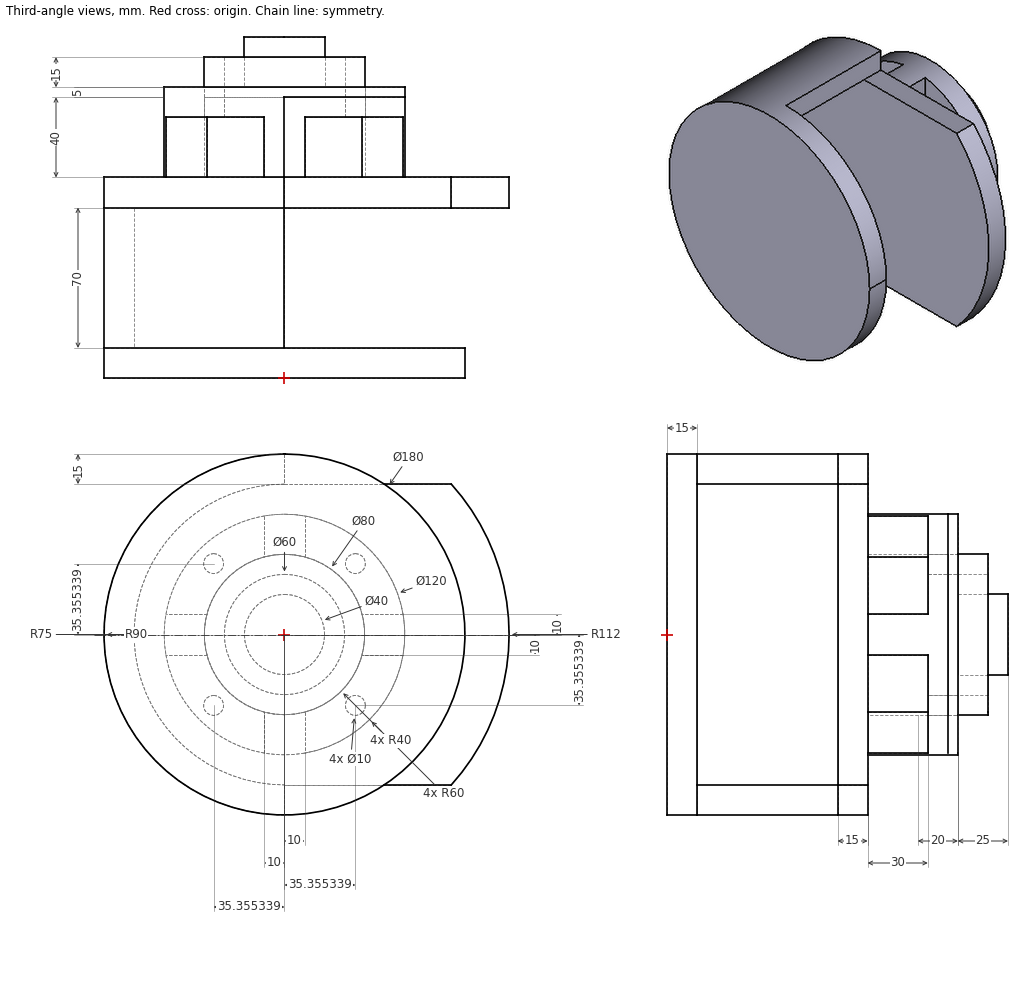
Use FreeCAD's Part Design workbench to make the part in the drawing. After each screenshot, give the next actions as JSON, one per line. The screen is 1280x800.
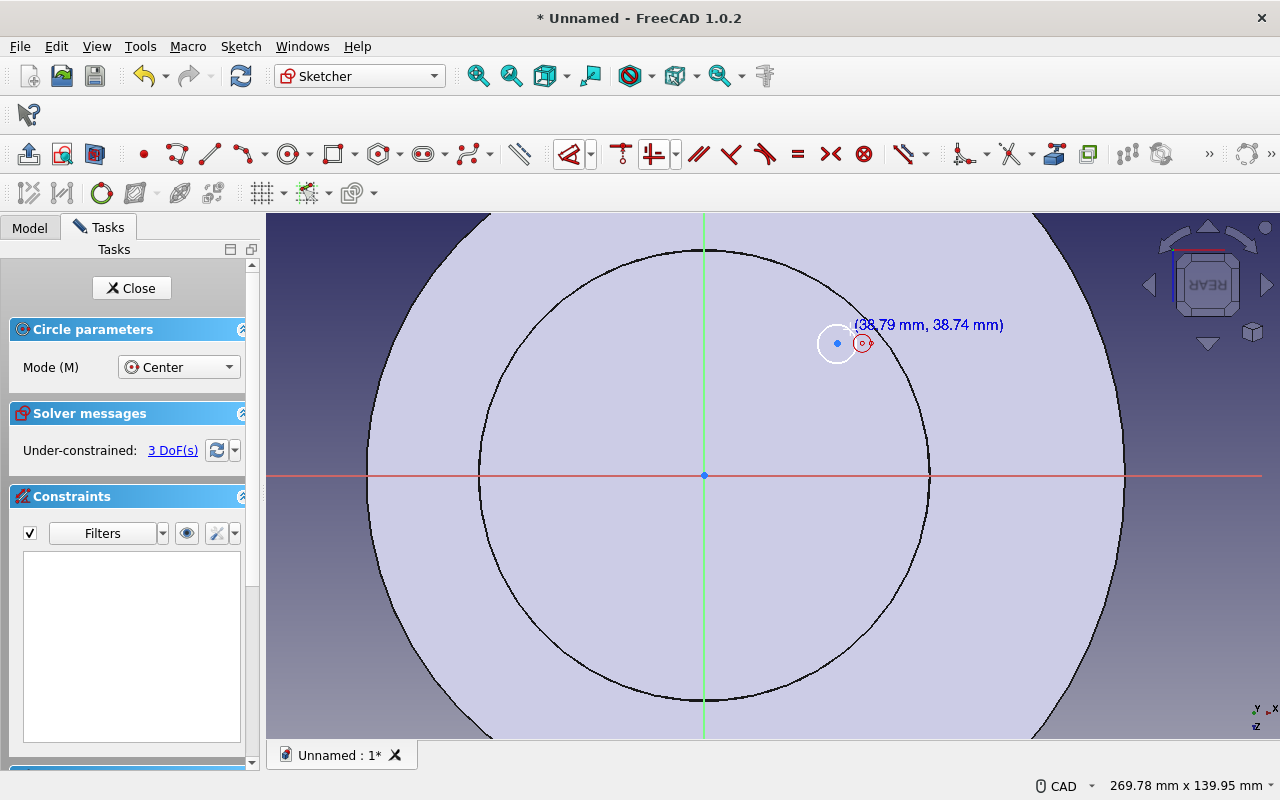
{"action": "left_click", "coordinate": [571, 343]}
{"action": "left_click", "coordinate": [585, 329]}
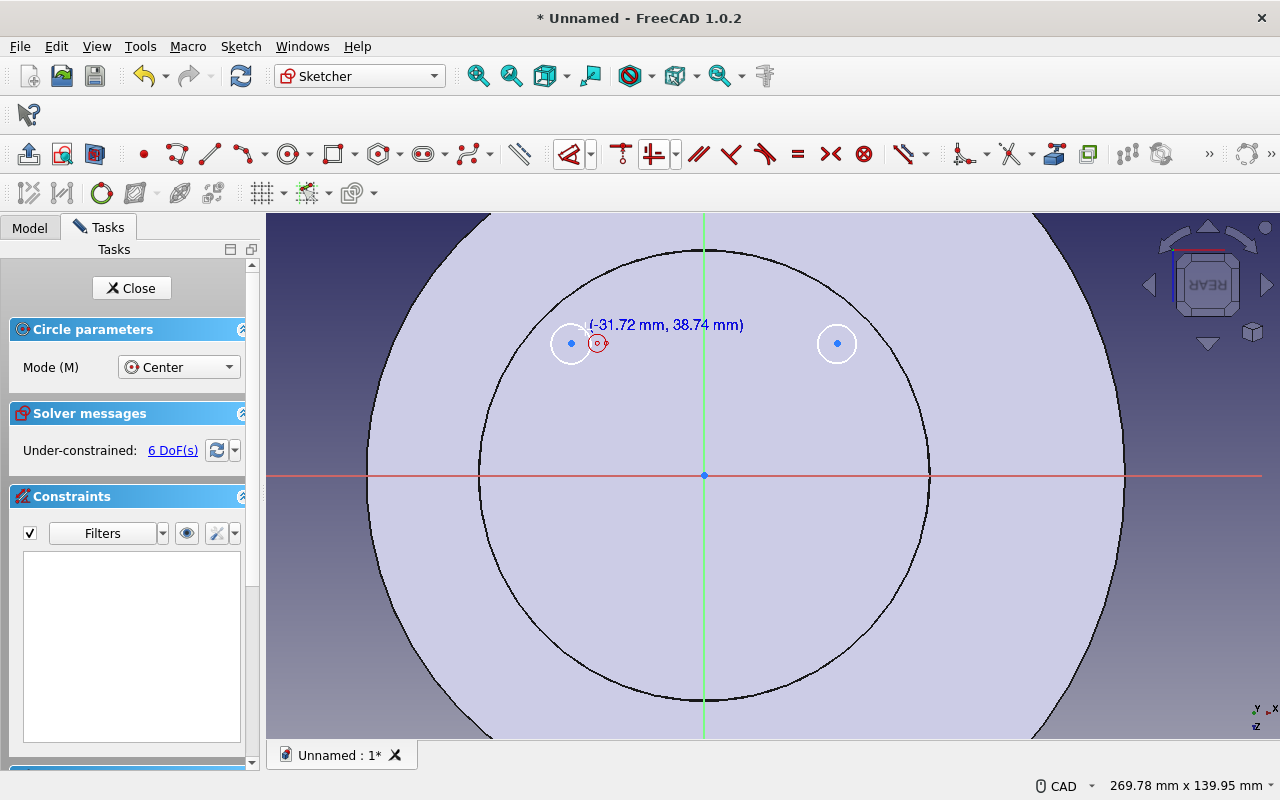
{"action": "left_click", "coordinate": [571, 608]}
{"action": "left_click", "coordinate": [585, 595]}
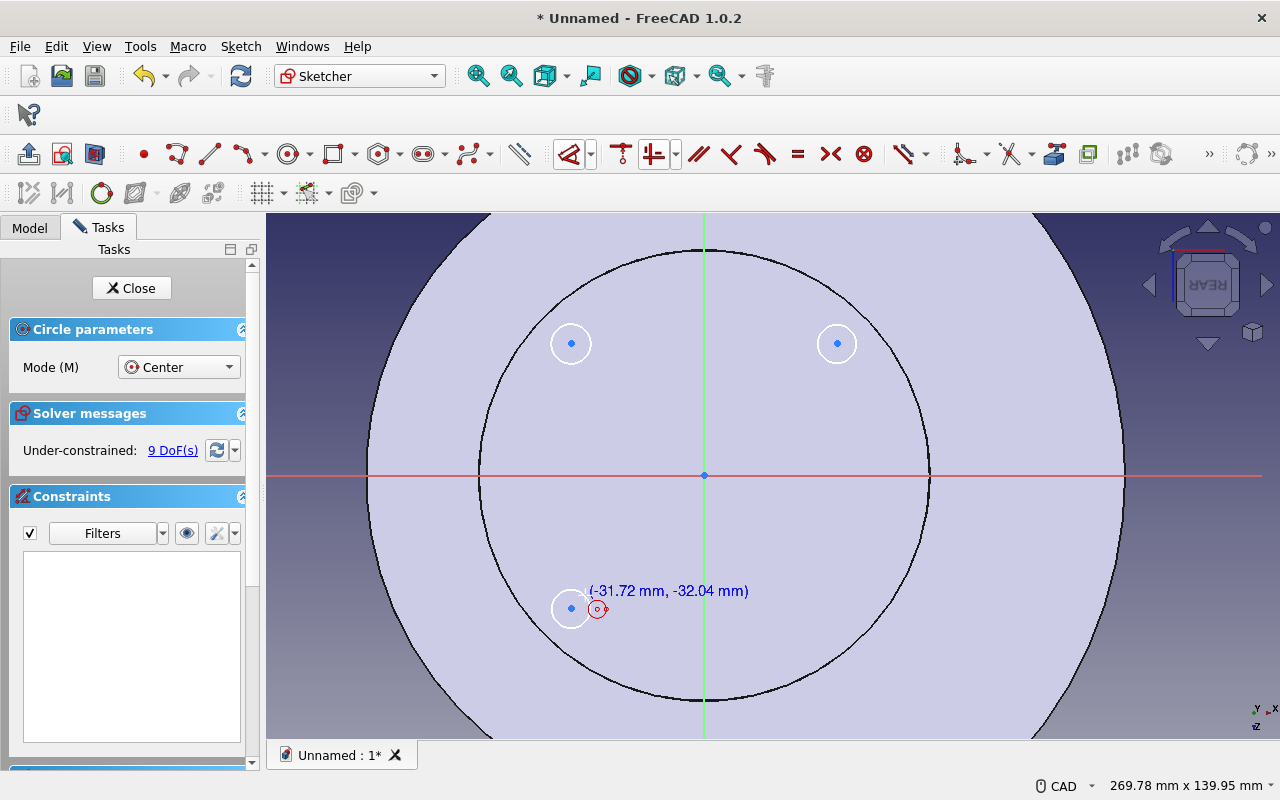
{"action": "left_click", "coordinate": [837, 608]}
{"action": "left_click", "coordinate": [850, 595]}
{"action": "key", "text": "Escape"}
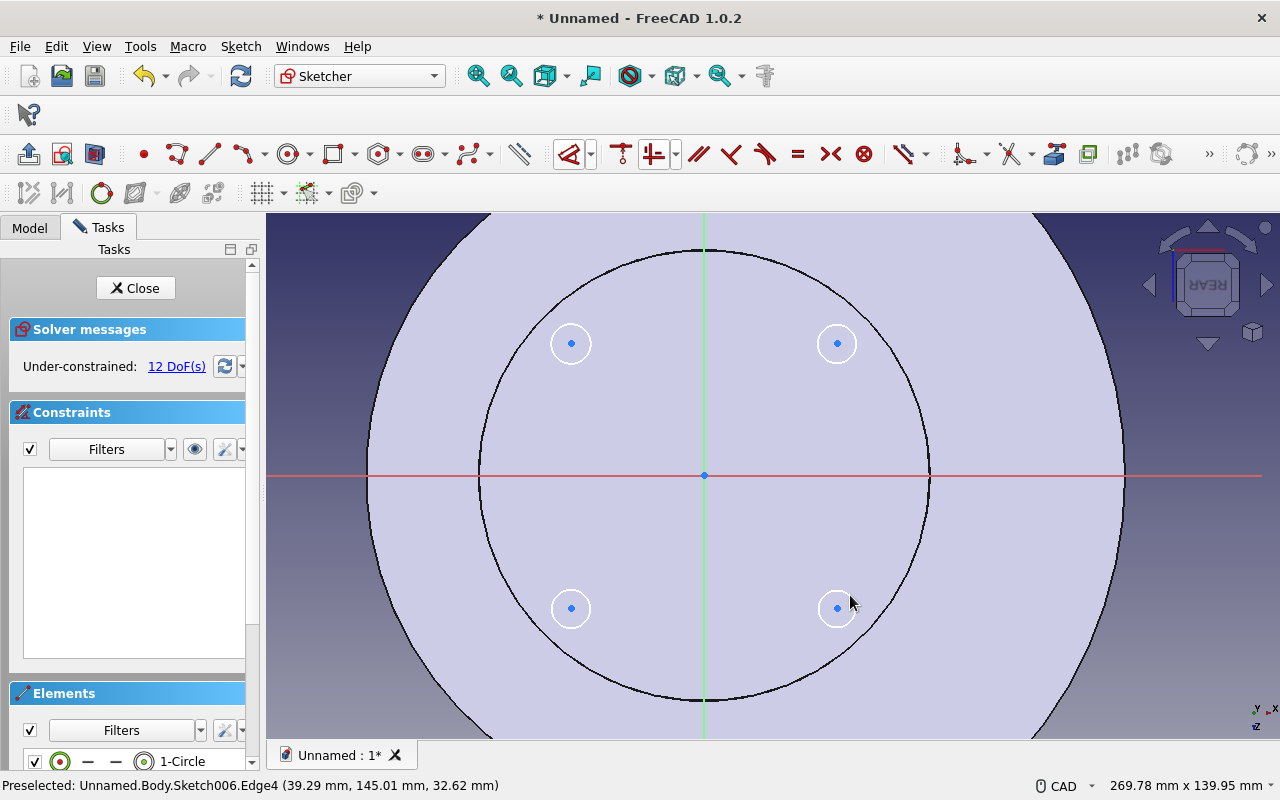
{"action": "left_click", "coordinate": [850, 330]}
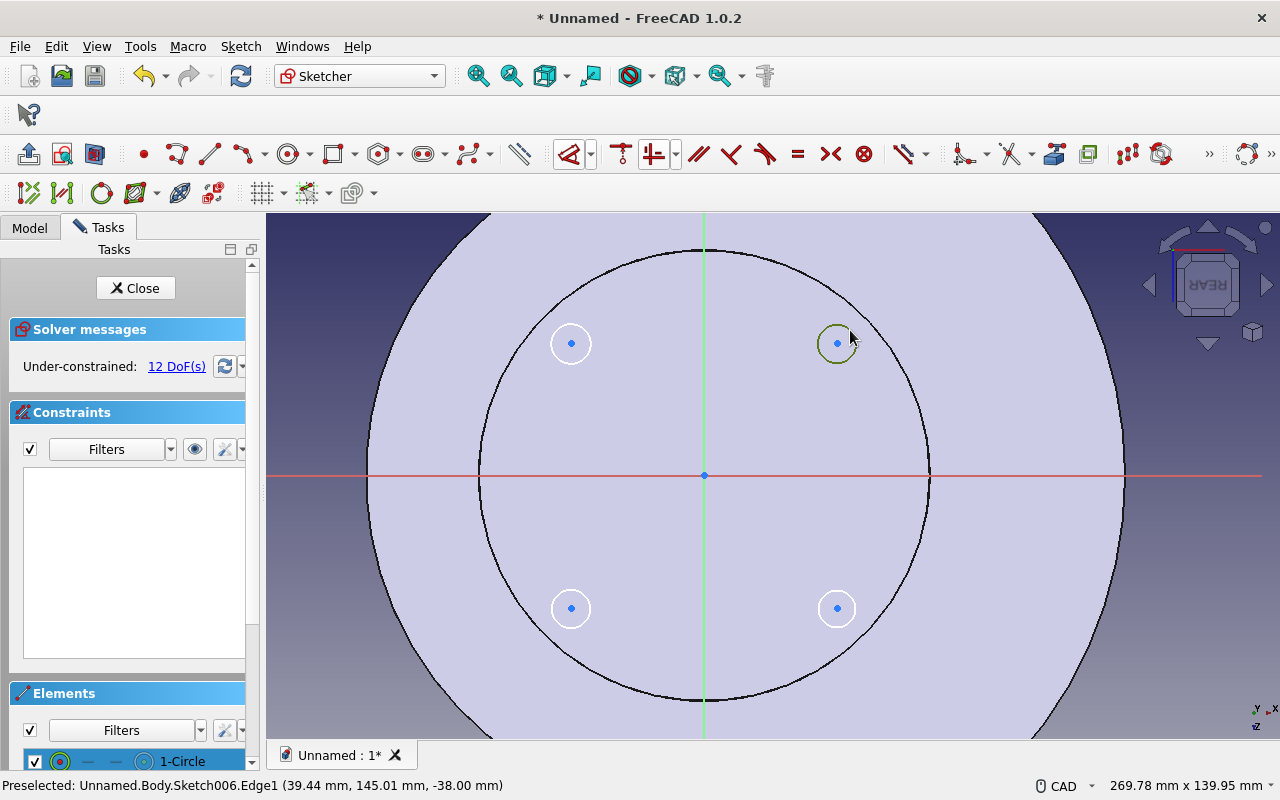
{"action": "left_click", "coordinate": [585, 330]}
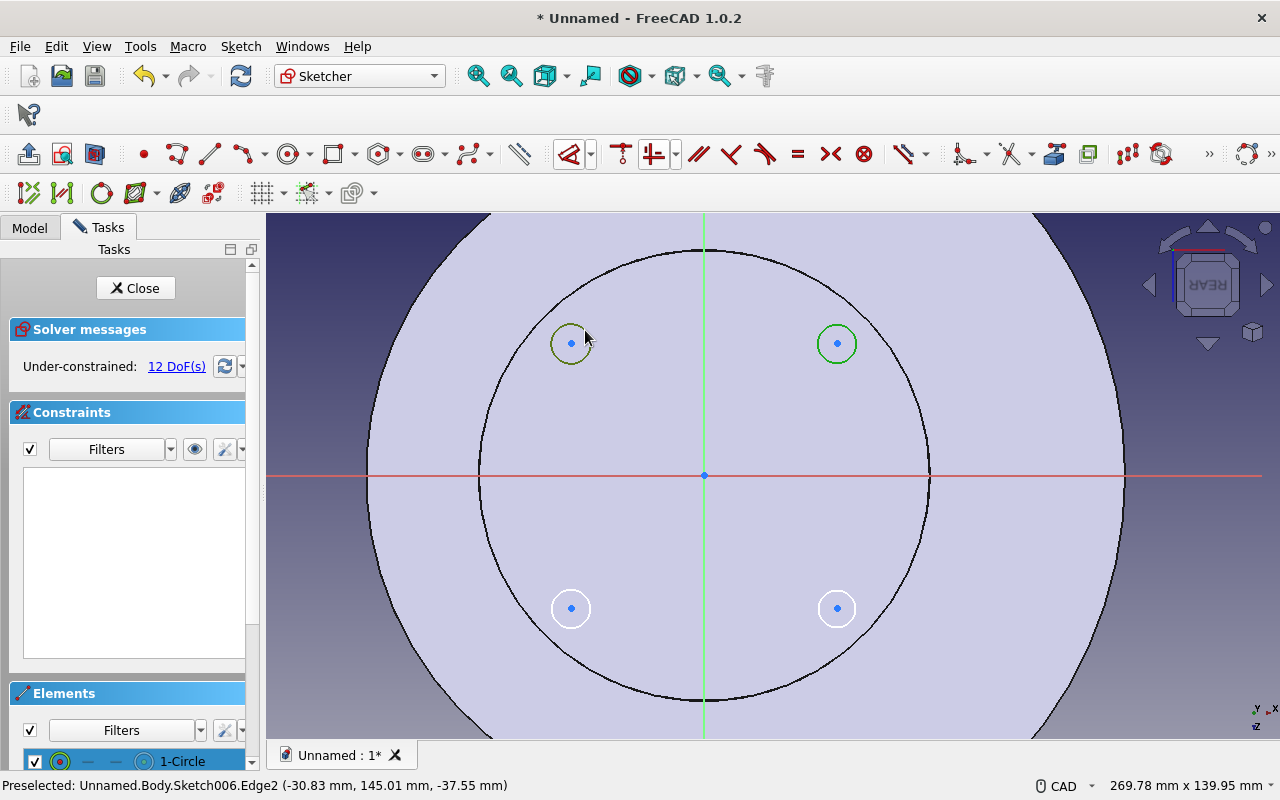
{"action": "left_click", "coordinate": [584, 595]}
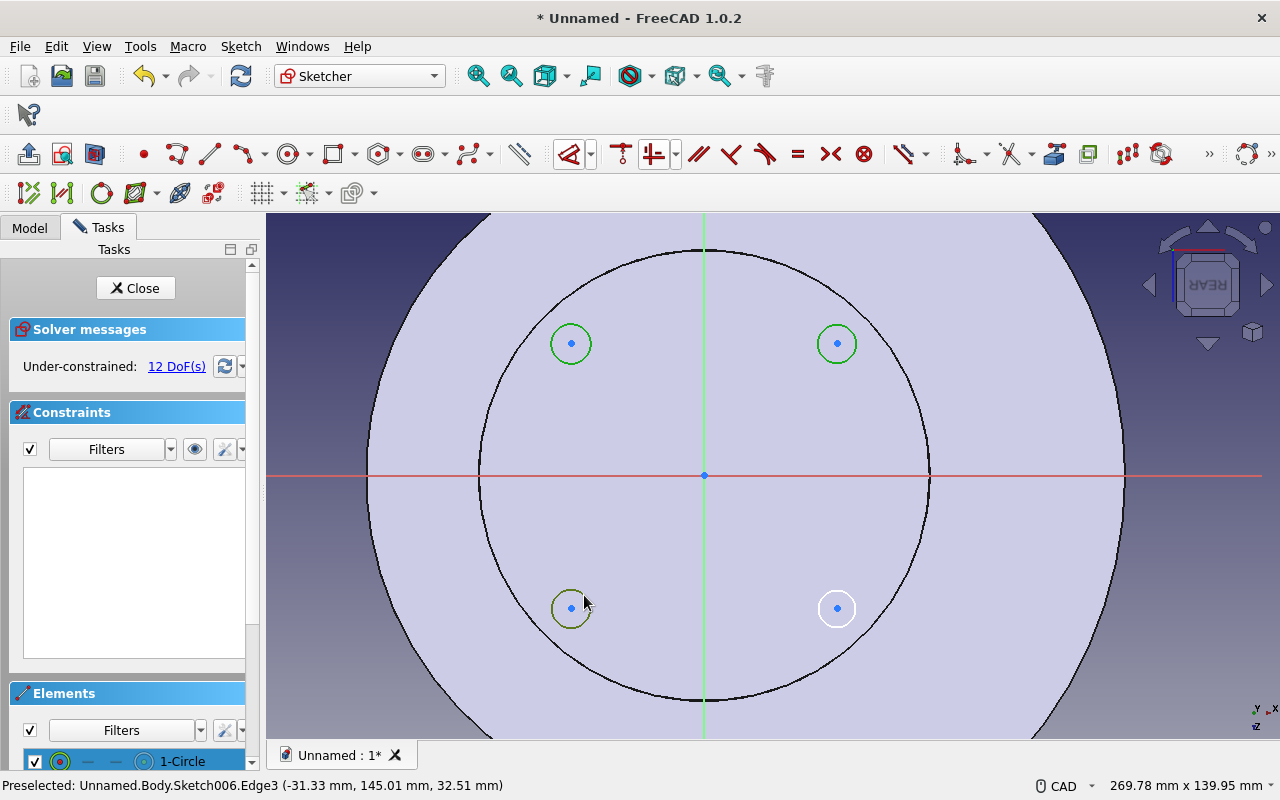
{"action": "left_click", "coordinate": [850, 596]}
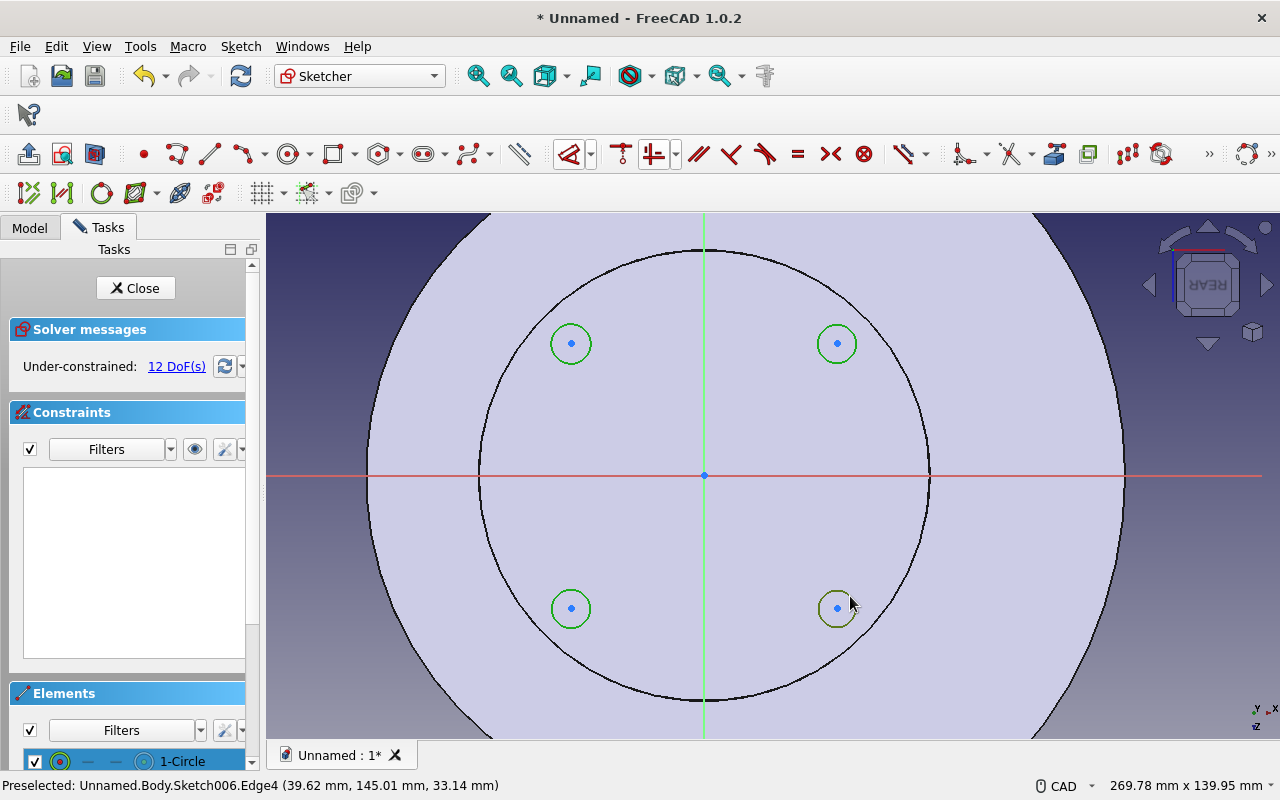
{"action": "left_click", "coordinate": [798, 154]}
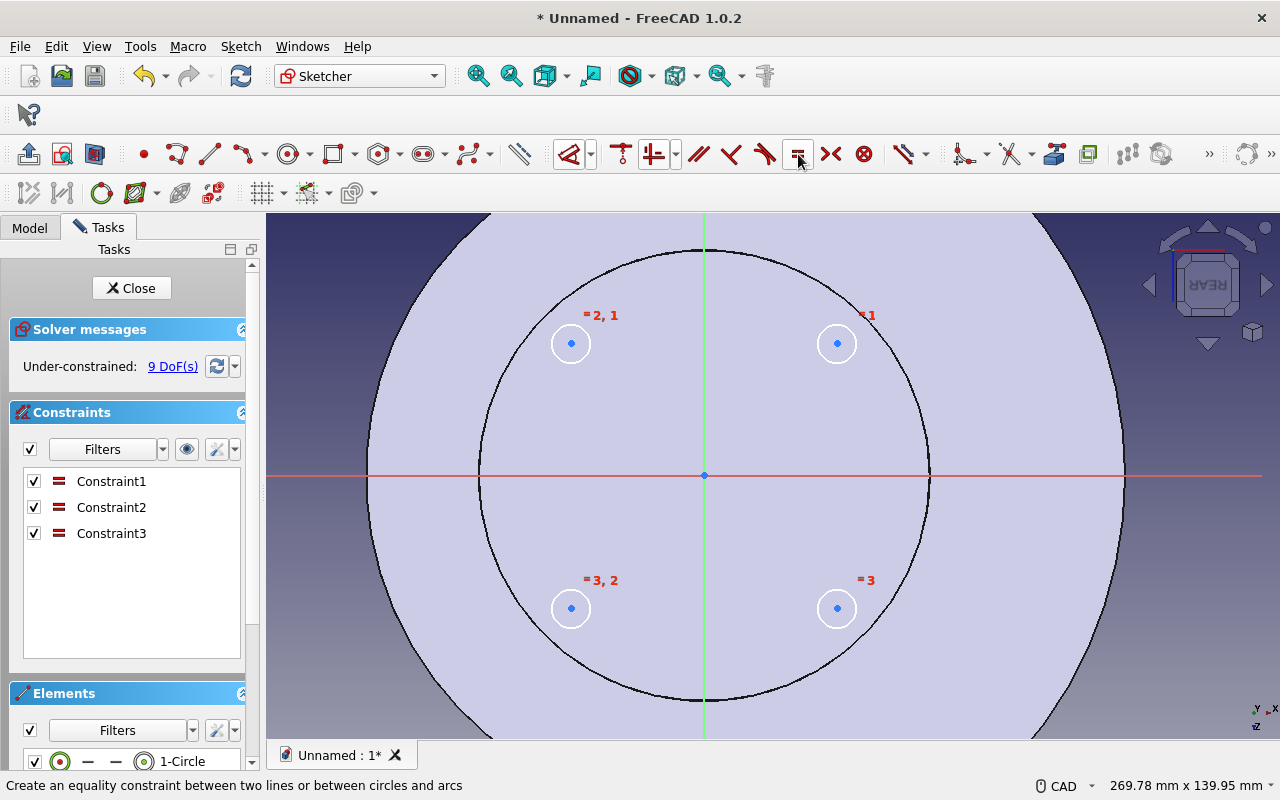
{"action": "left_click", "coordinate": [837, 344]}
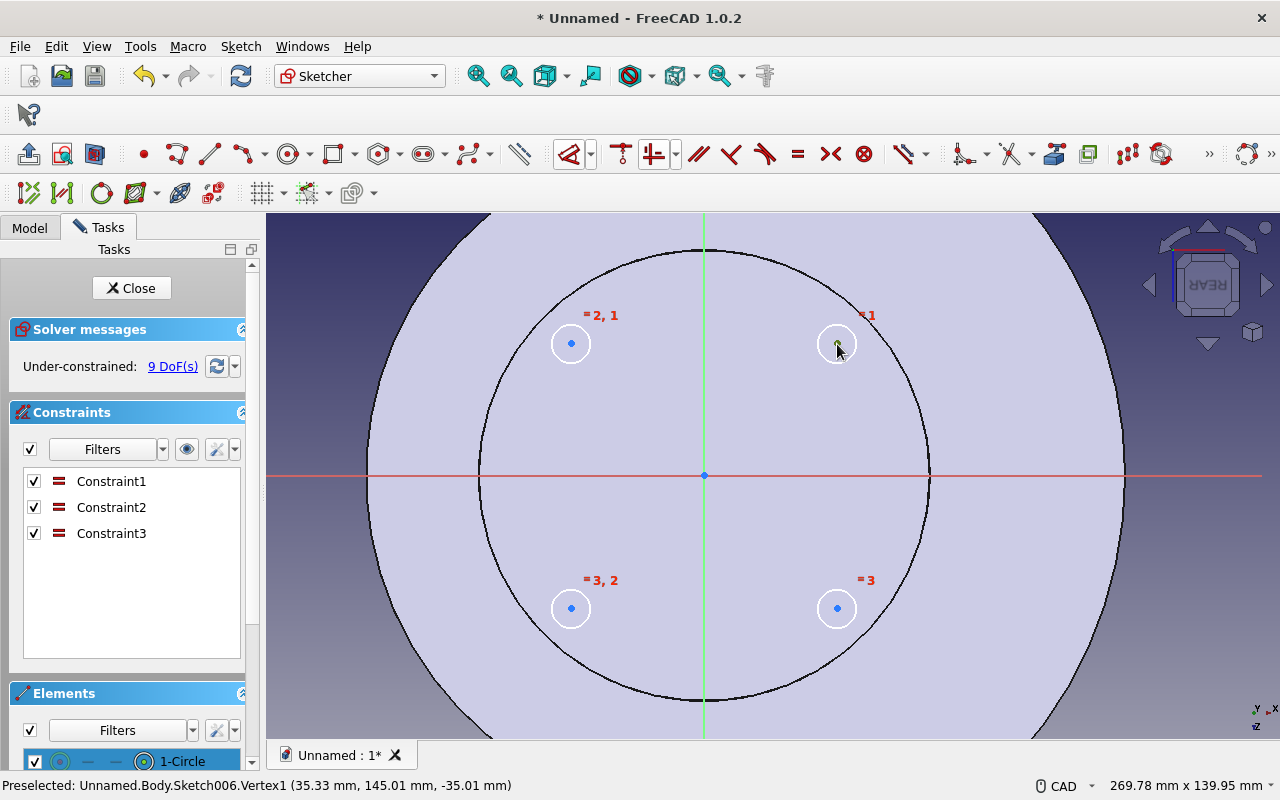
{"action": "left_click", "coordinate": [571, 344]}